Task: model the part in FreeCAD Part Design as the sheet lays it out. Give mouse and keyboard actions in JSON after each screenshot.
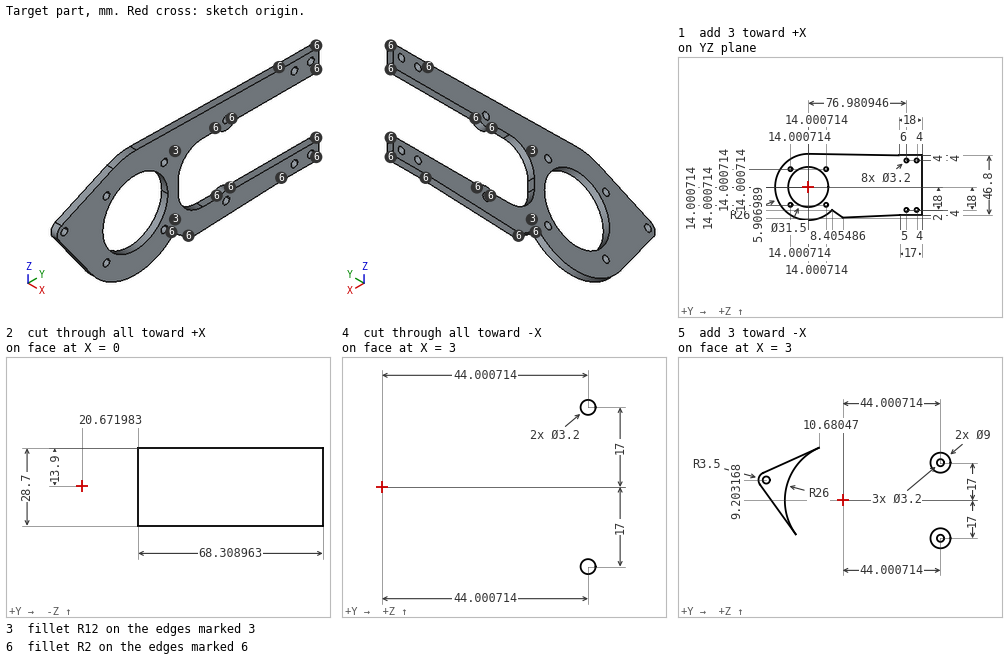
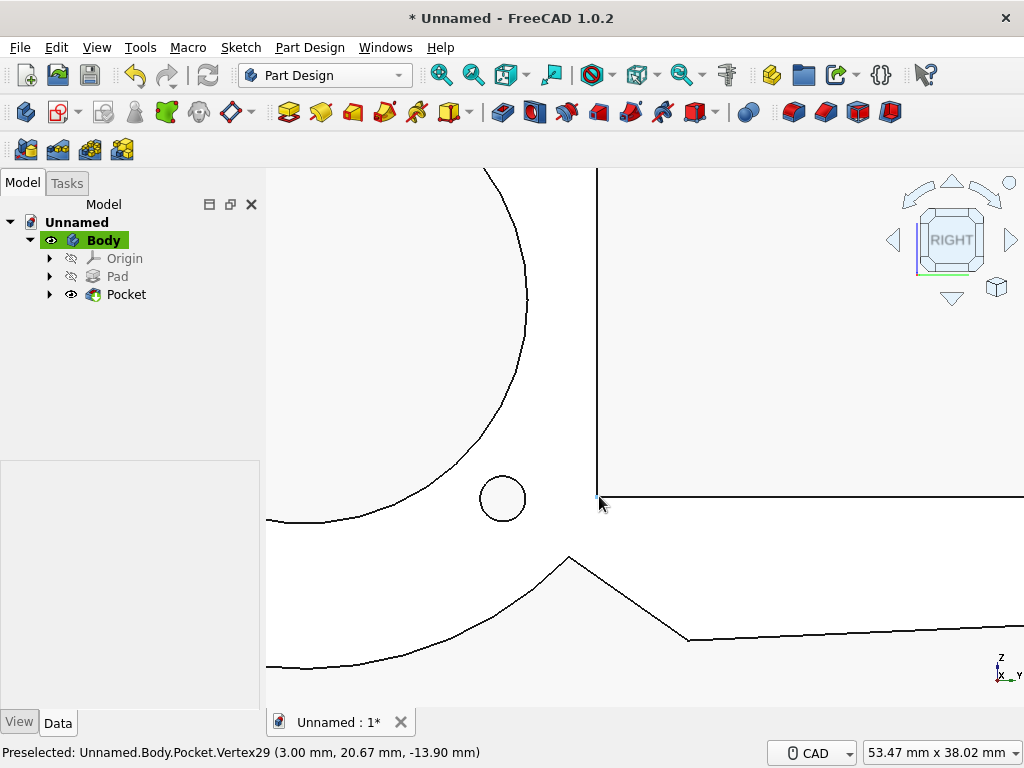
{"action": "left_click", "coordinate": [442, 76]}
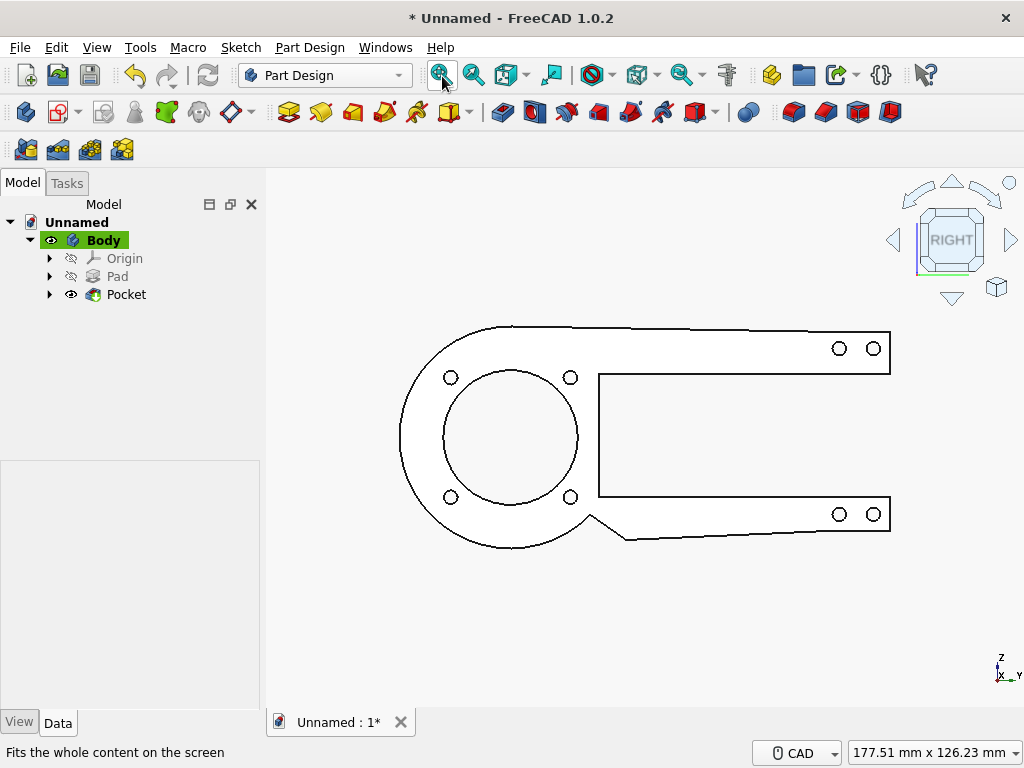
{"action": "key", "text": "5"}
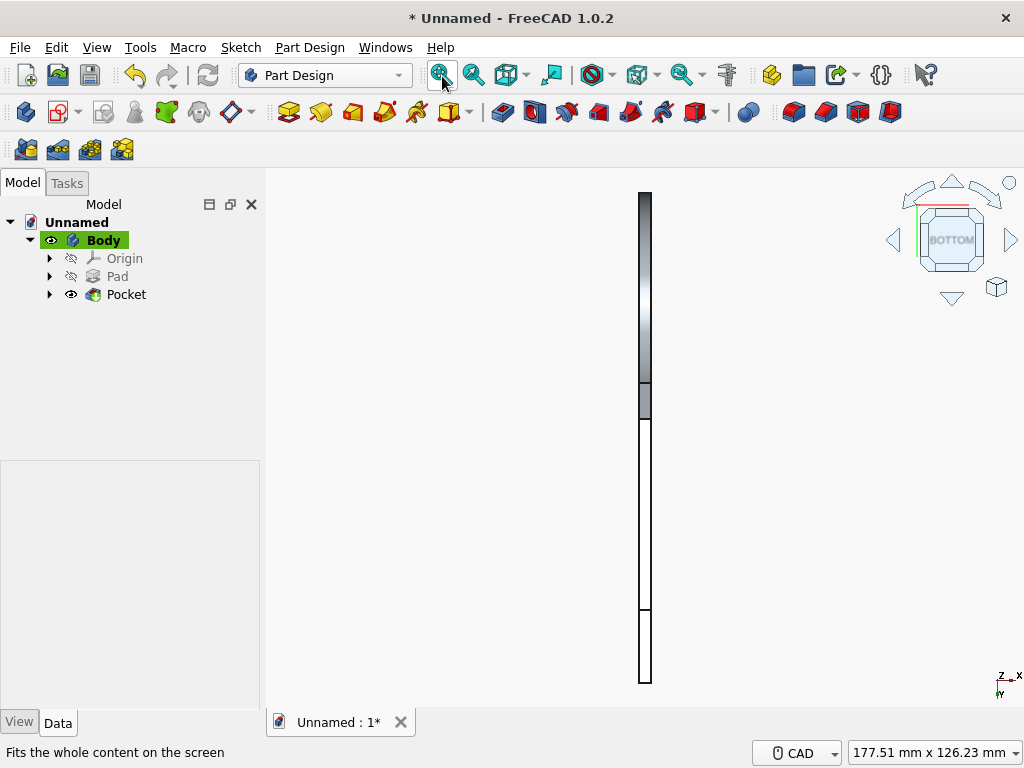
{"action": "scroll", "coordinate": [645, 390], "scroll_direction": "up", "scroll_amount": 6}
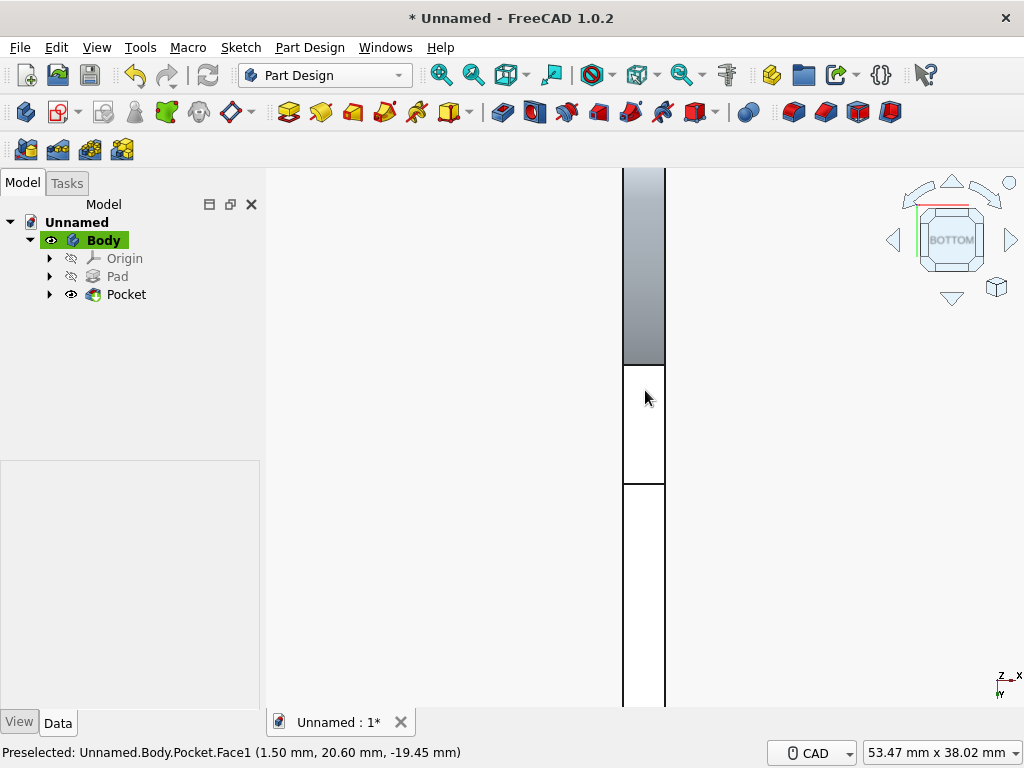
{"action": "left_click", "coordinate": [442, 76]}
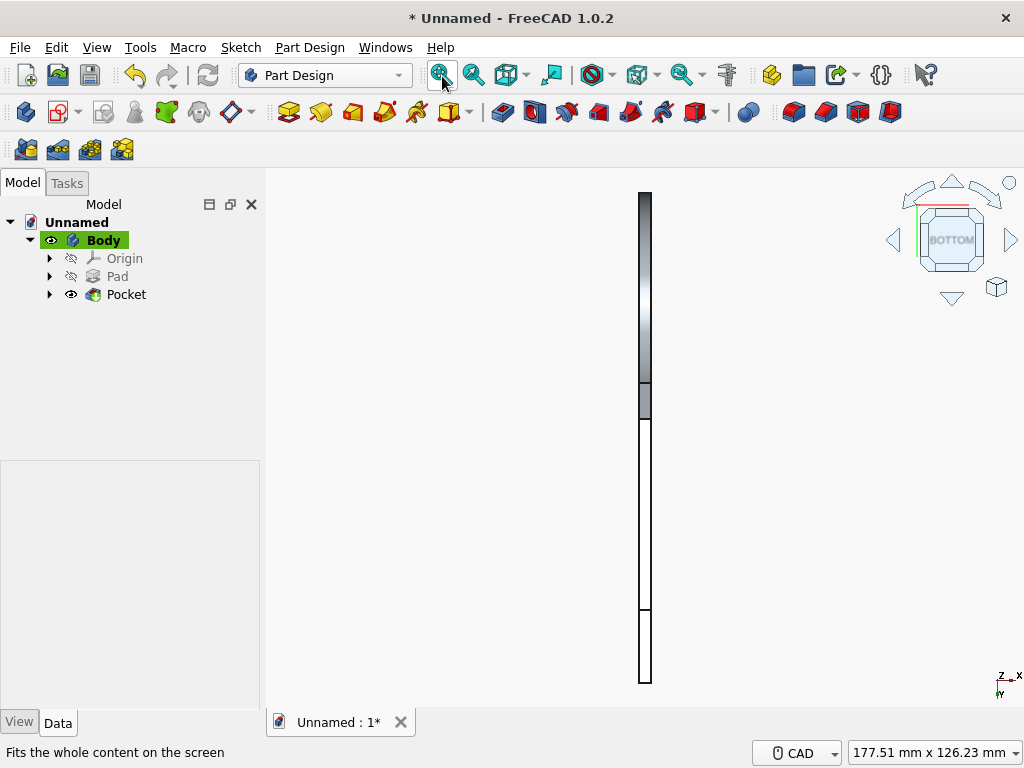
{"action": "key", "text": "4"}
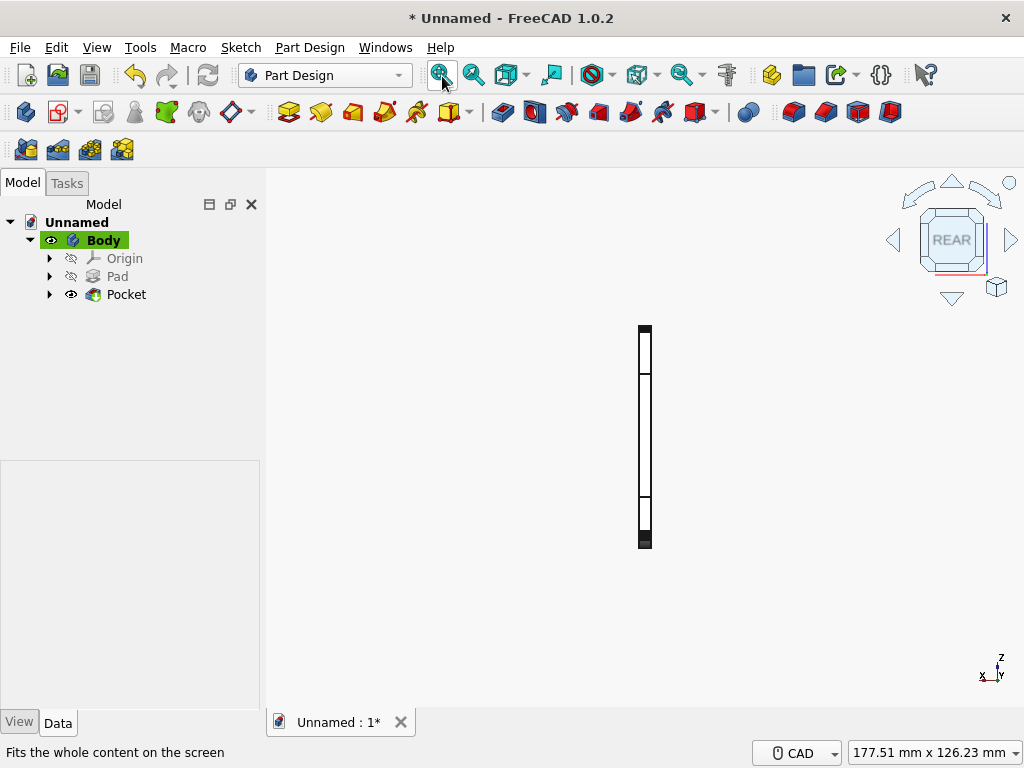
{"action": "left_click", "coordinate": [442, 76]}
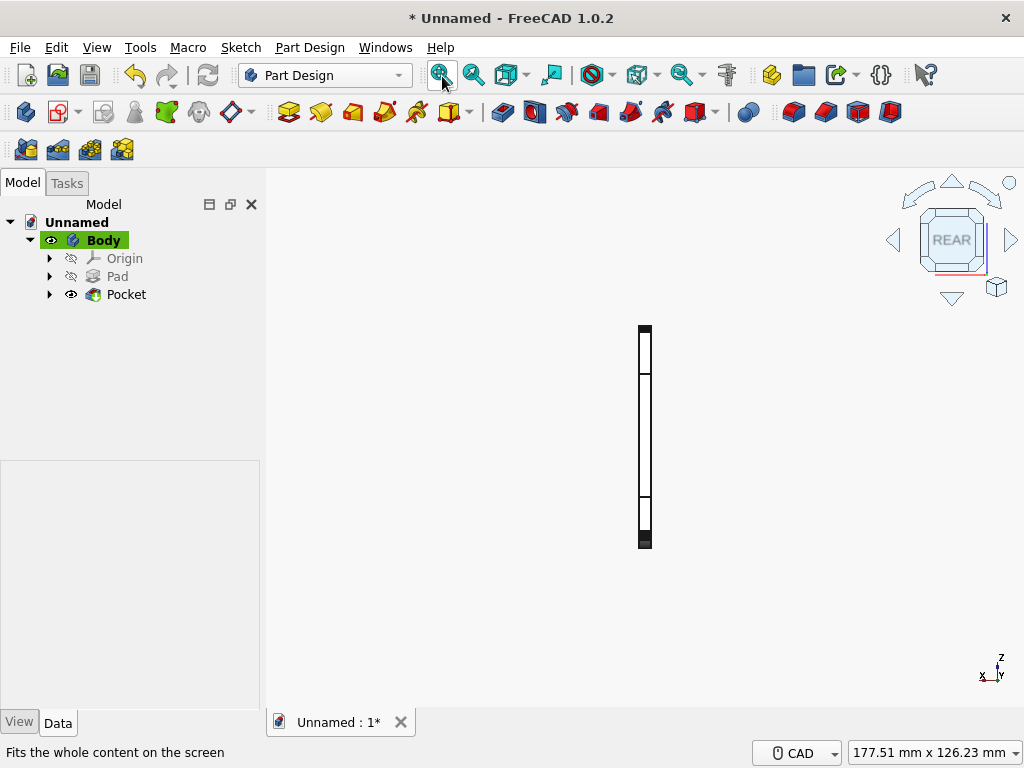
{"action": "scroll", "coordinate": [645, 496], "scroll_direction": "up", "scroll_amount": 6}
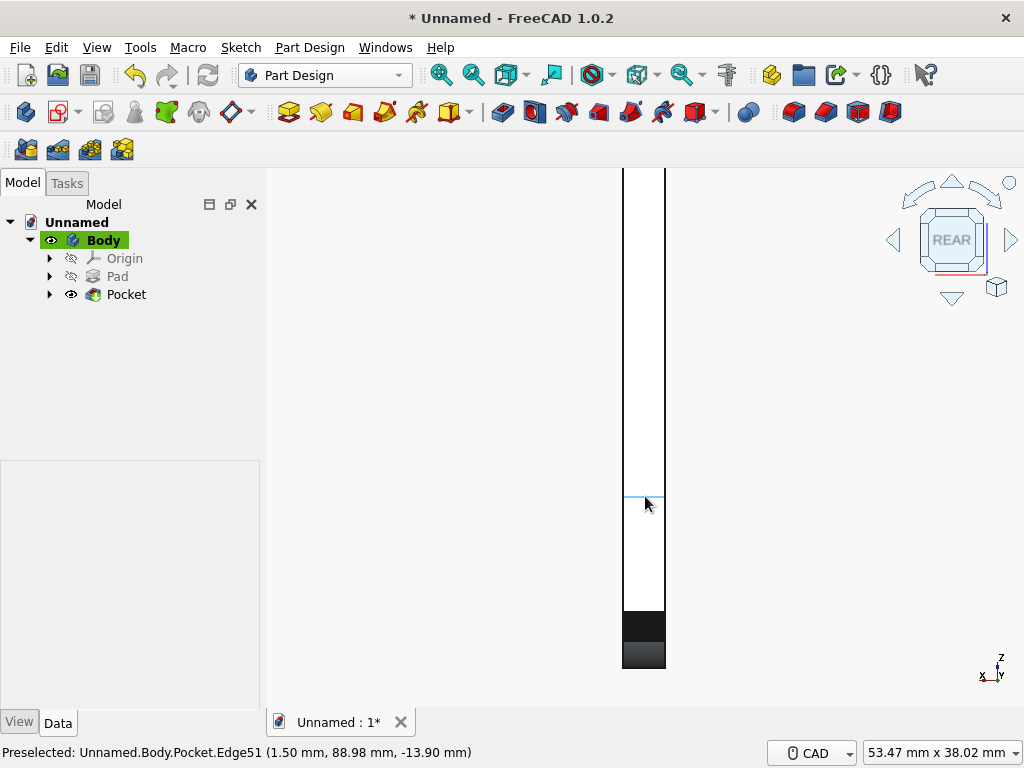
{"action": "left_click", "coordinate": [442, 76]}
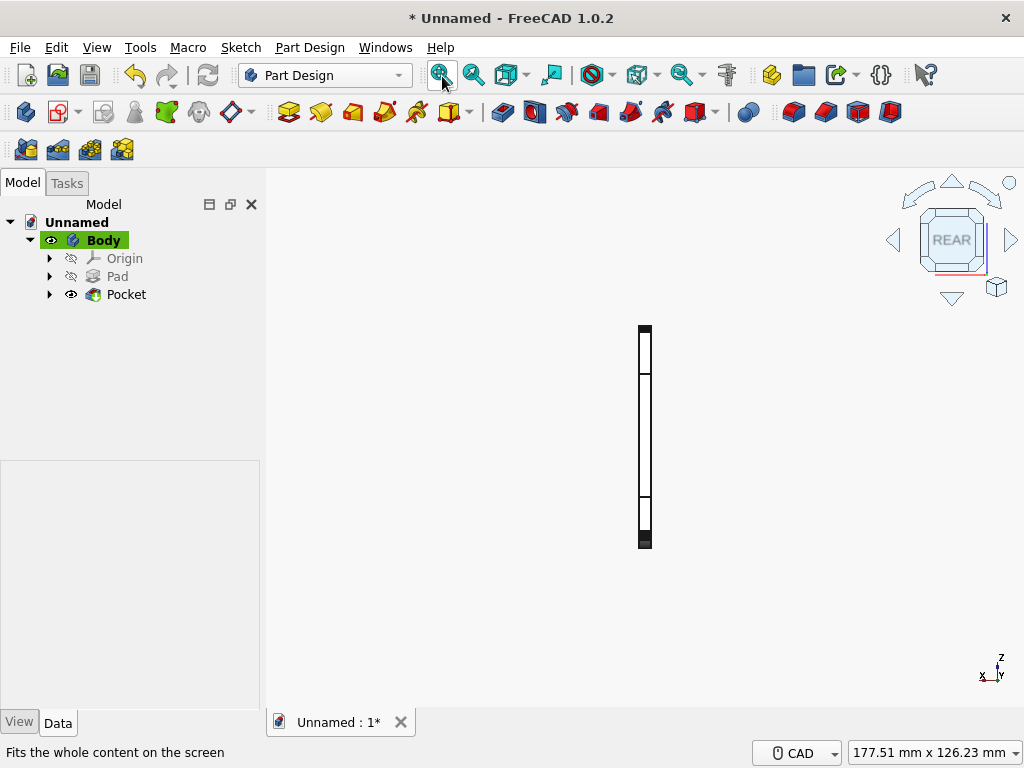
{"action": "key", "text": "6"}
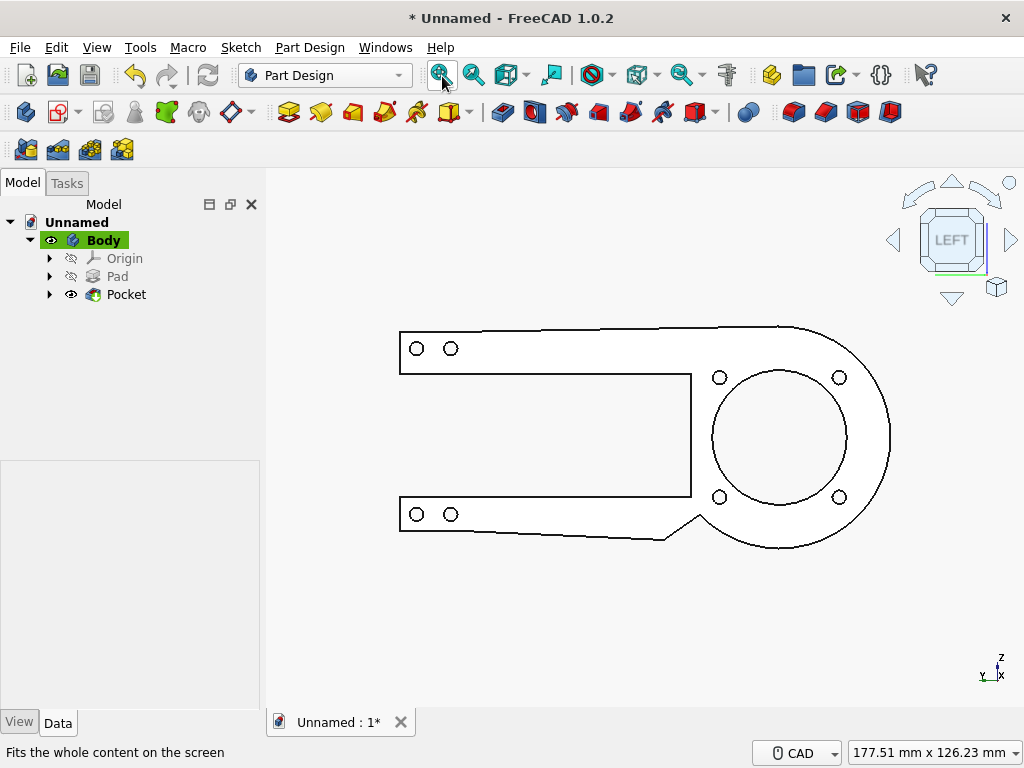
{"action": "scroll", "coordinate": [691, 496], "scroll_direction": "up", "scroll_amount": 6}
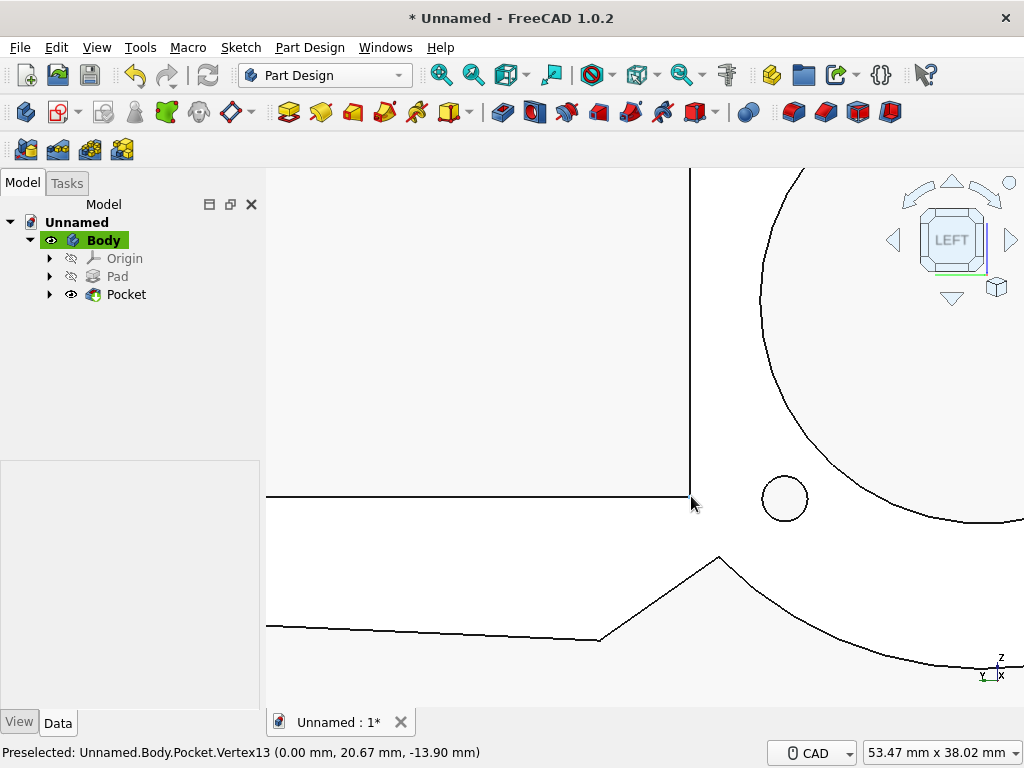
{"action": "left_click", "coordinate": [442, 76]}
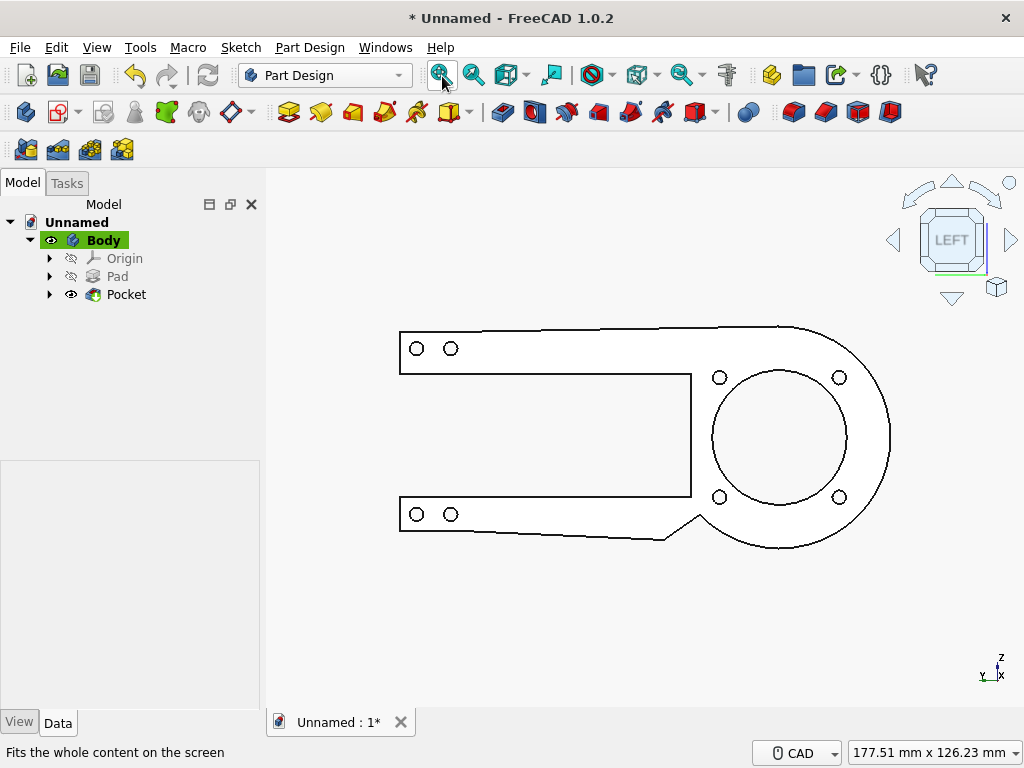
{"action": "key", "text": "v 3"}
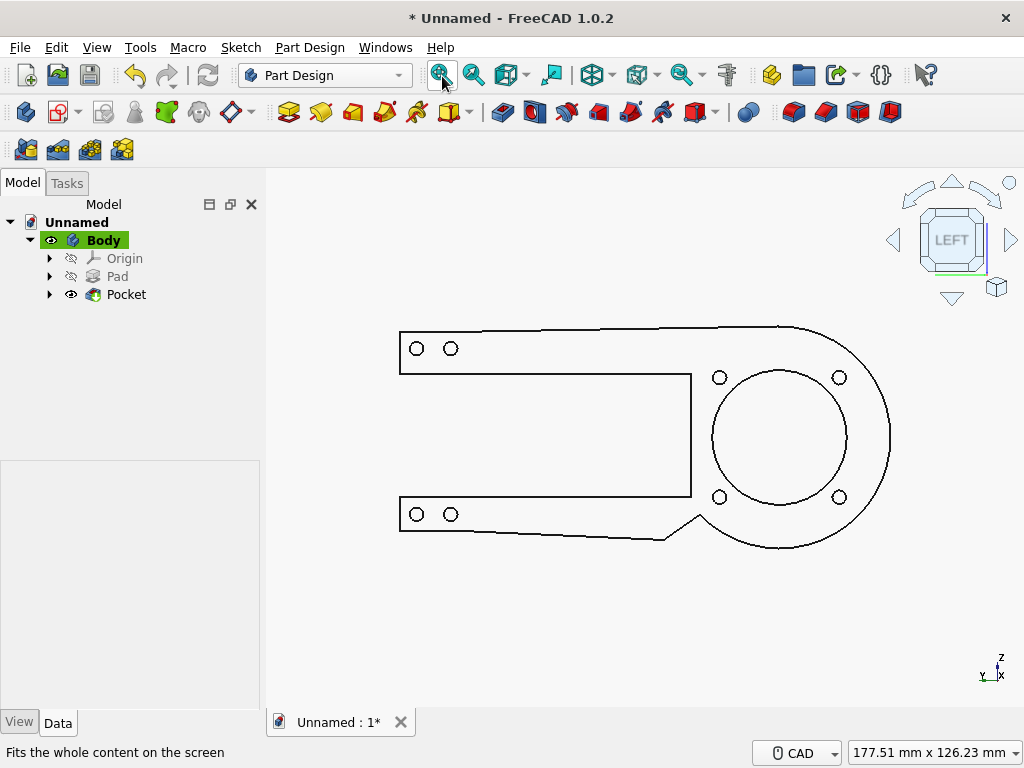
{"action": "key", "text": "0"}